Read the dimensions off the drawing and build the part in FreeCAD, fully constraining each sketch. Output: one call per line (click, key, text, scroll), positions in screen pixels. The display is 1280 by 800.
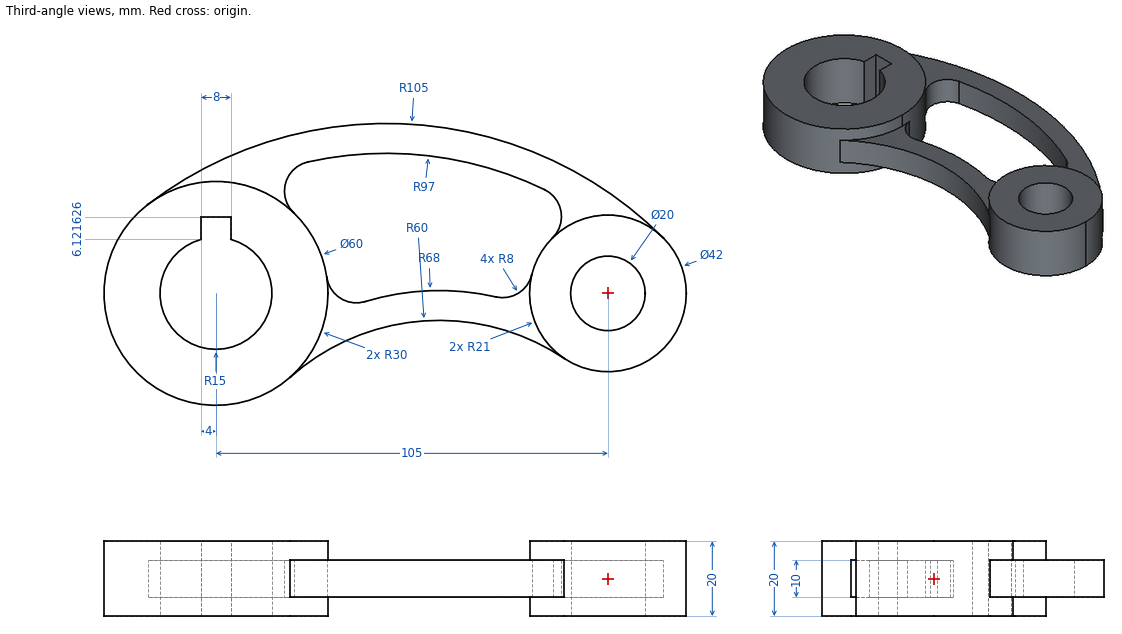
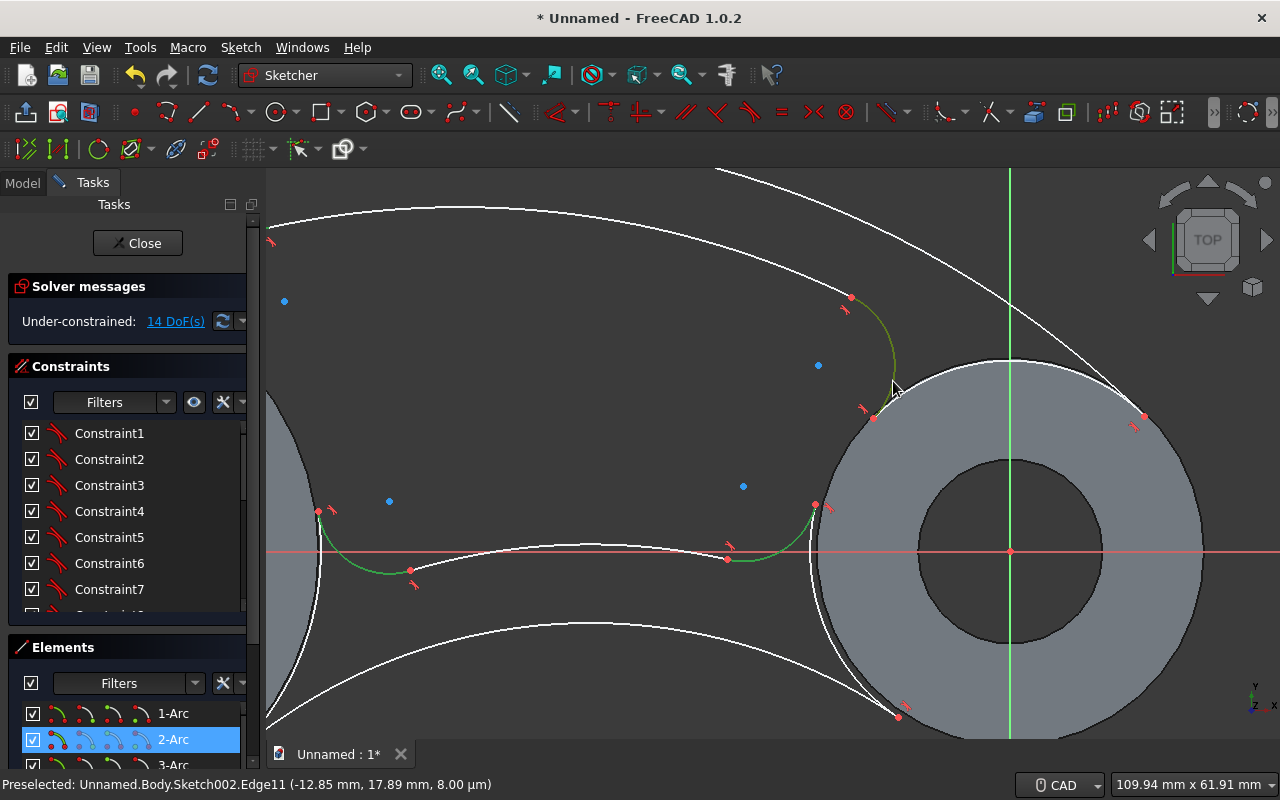
key(e)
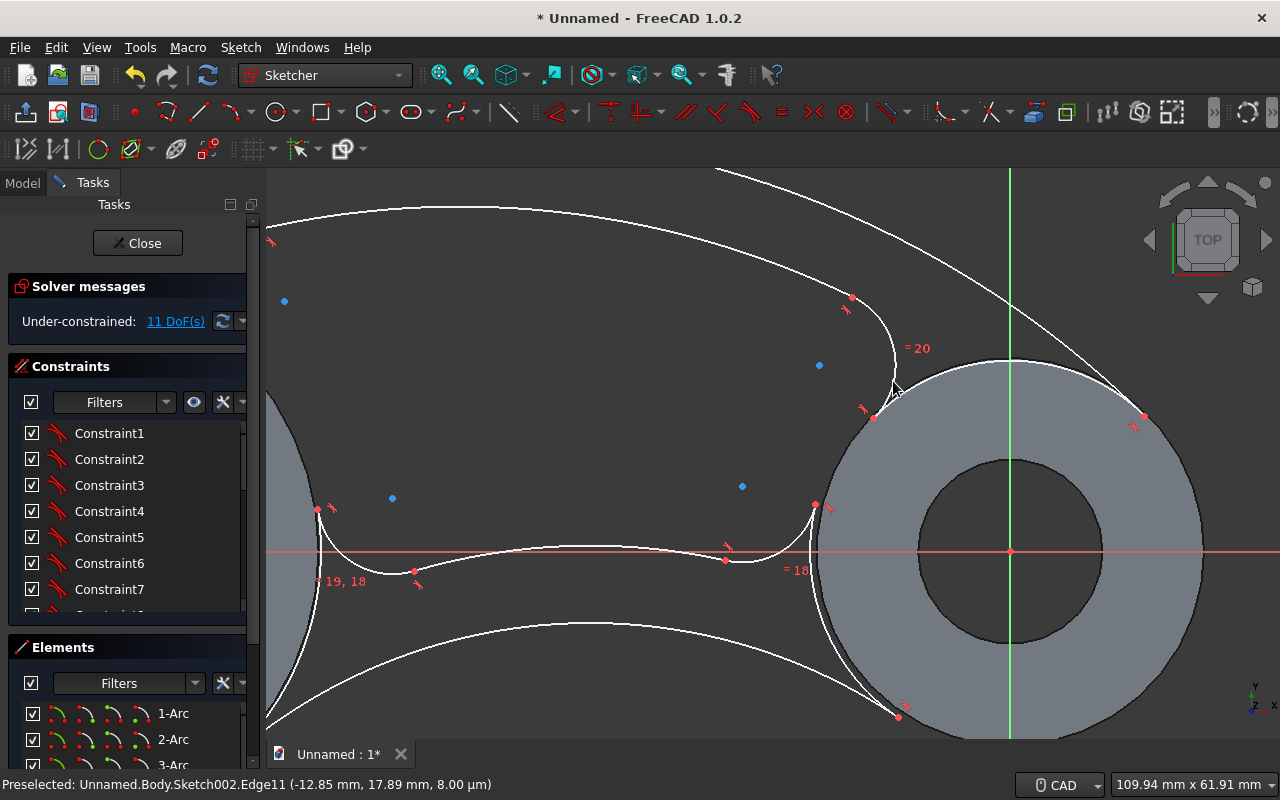
click(812, 577)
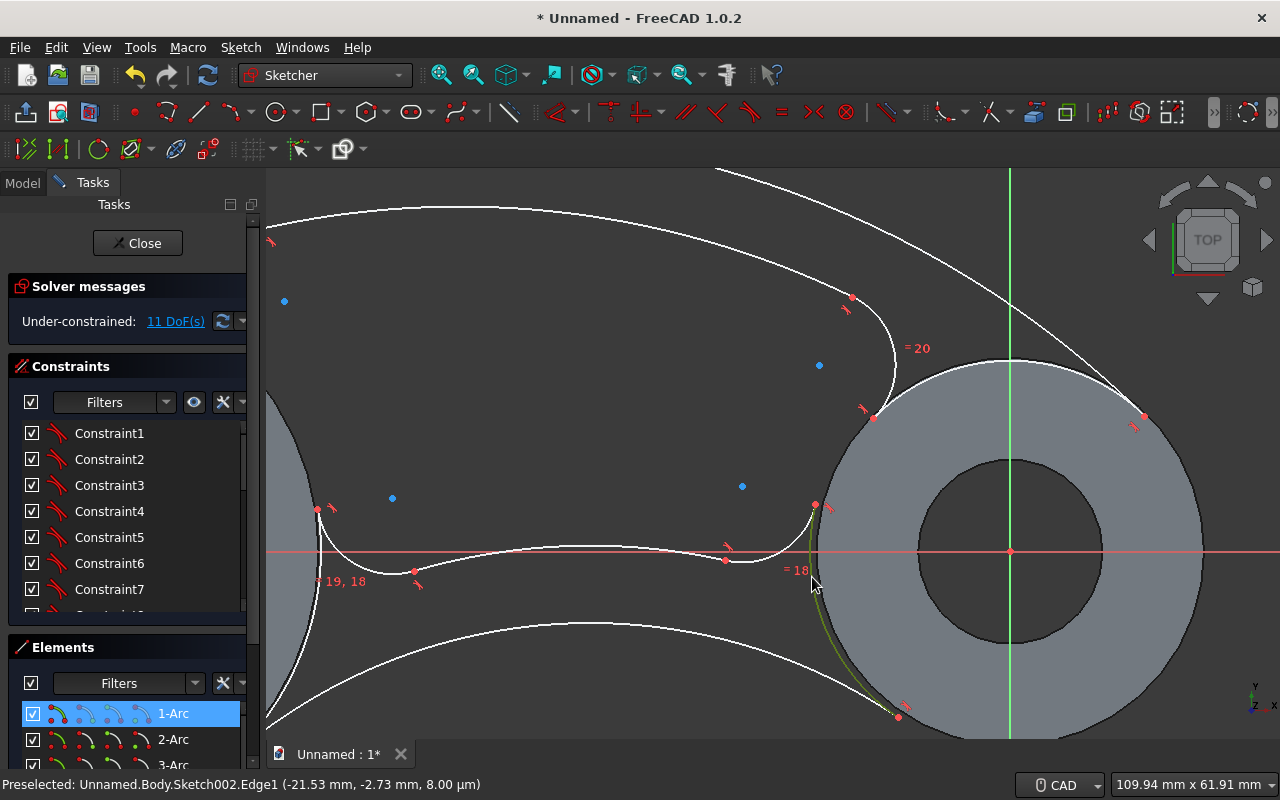
click(1068, 370)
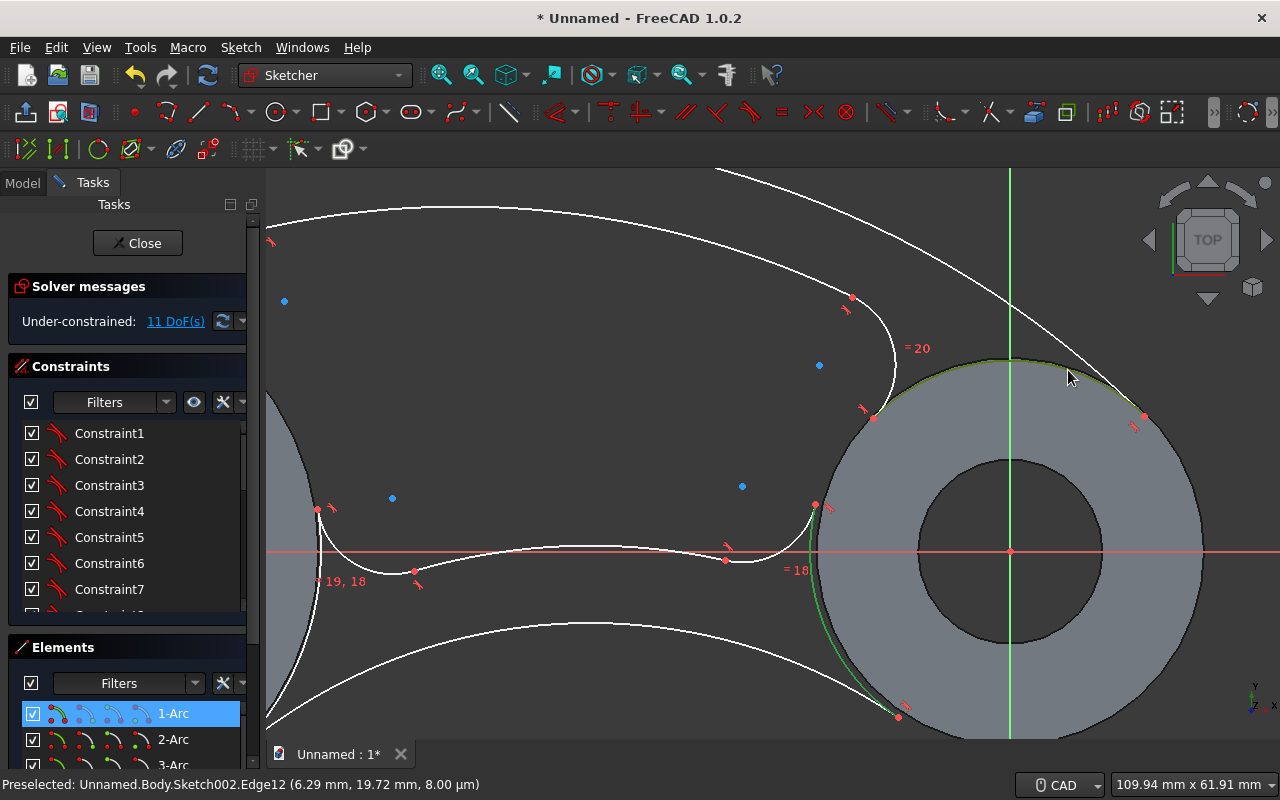
click(782, 112)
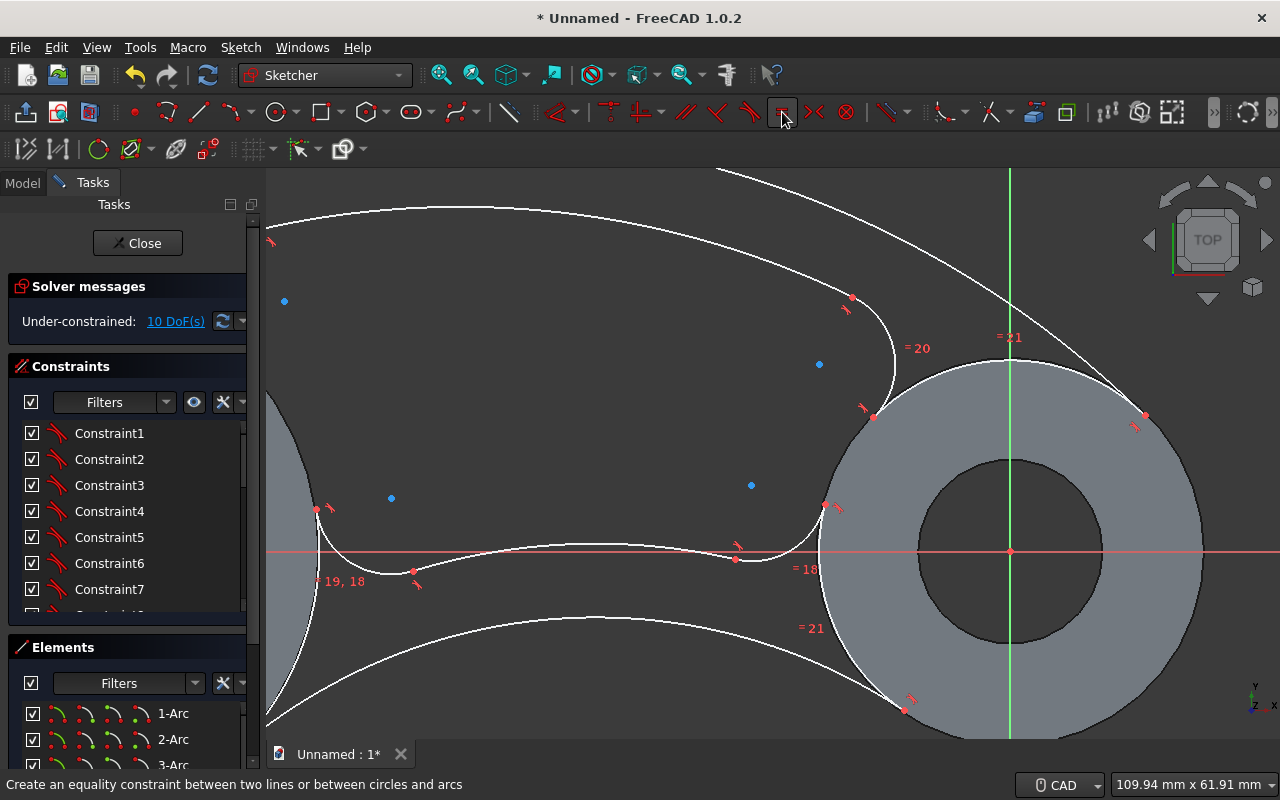
scroll(863, 460, down, 4)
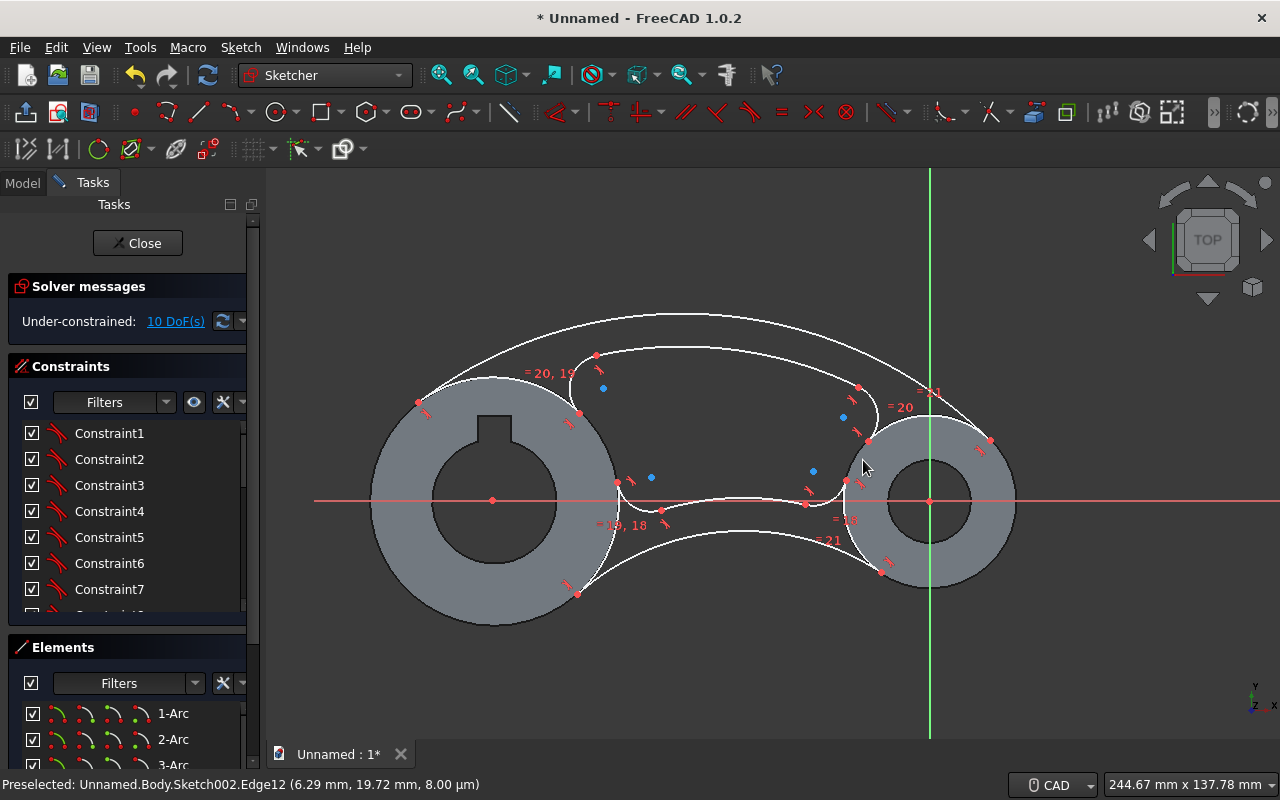
click(493, 501)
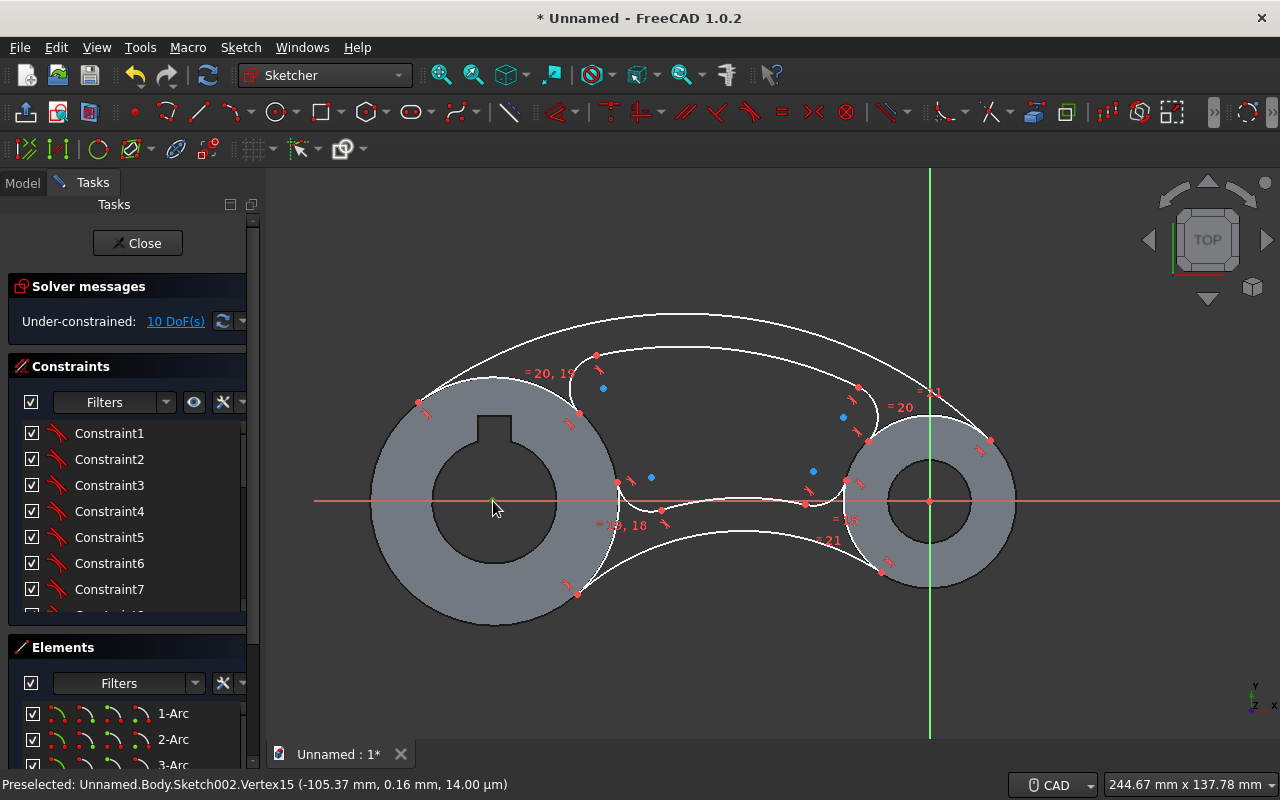
click(353, 501)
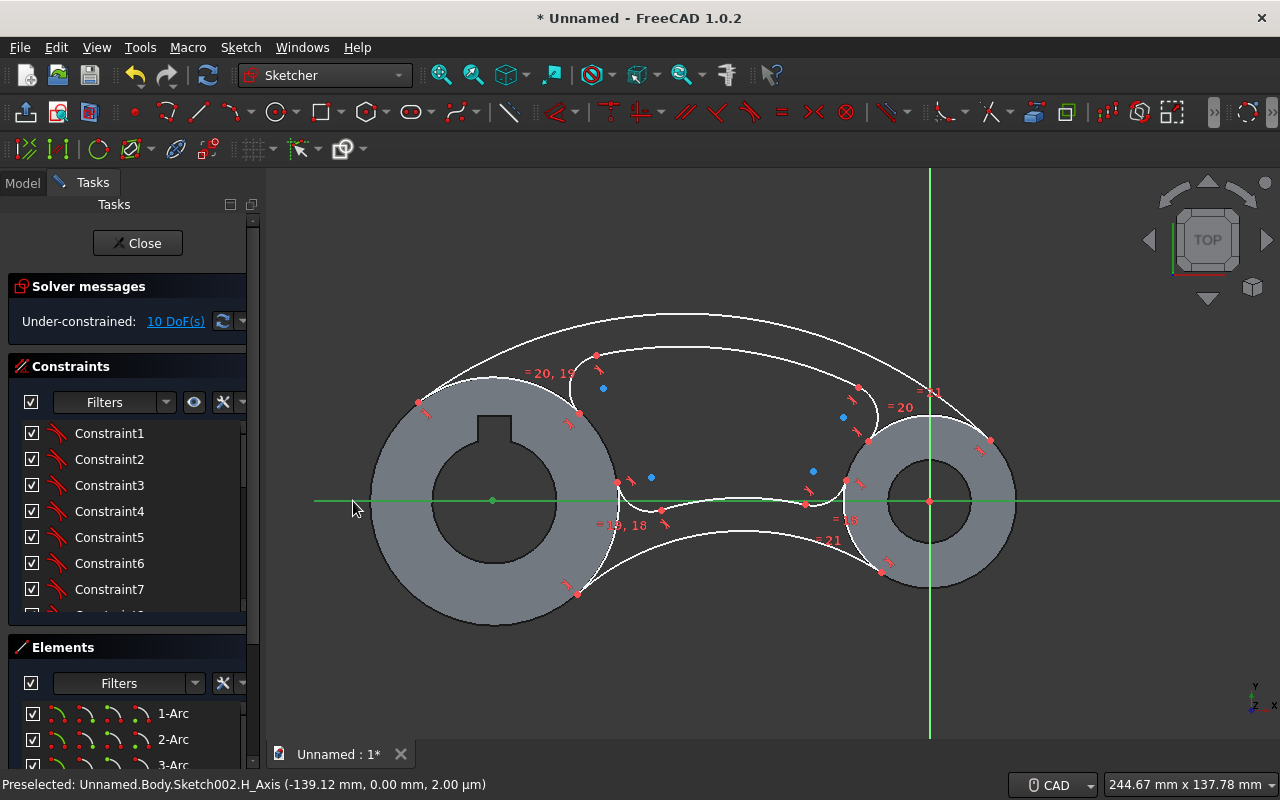
click(610, 112)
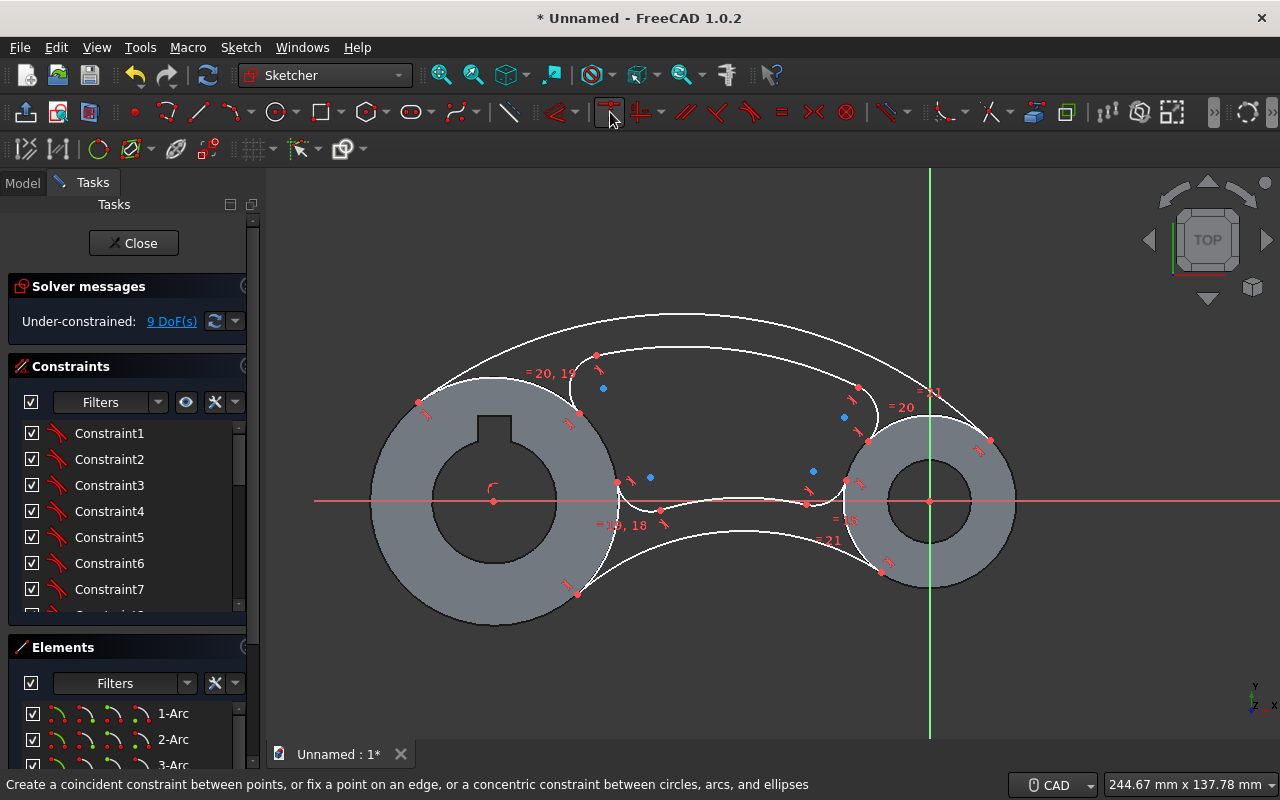
key(d)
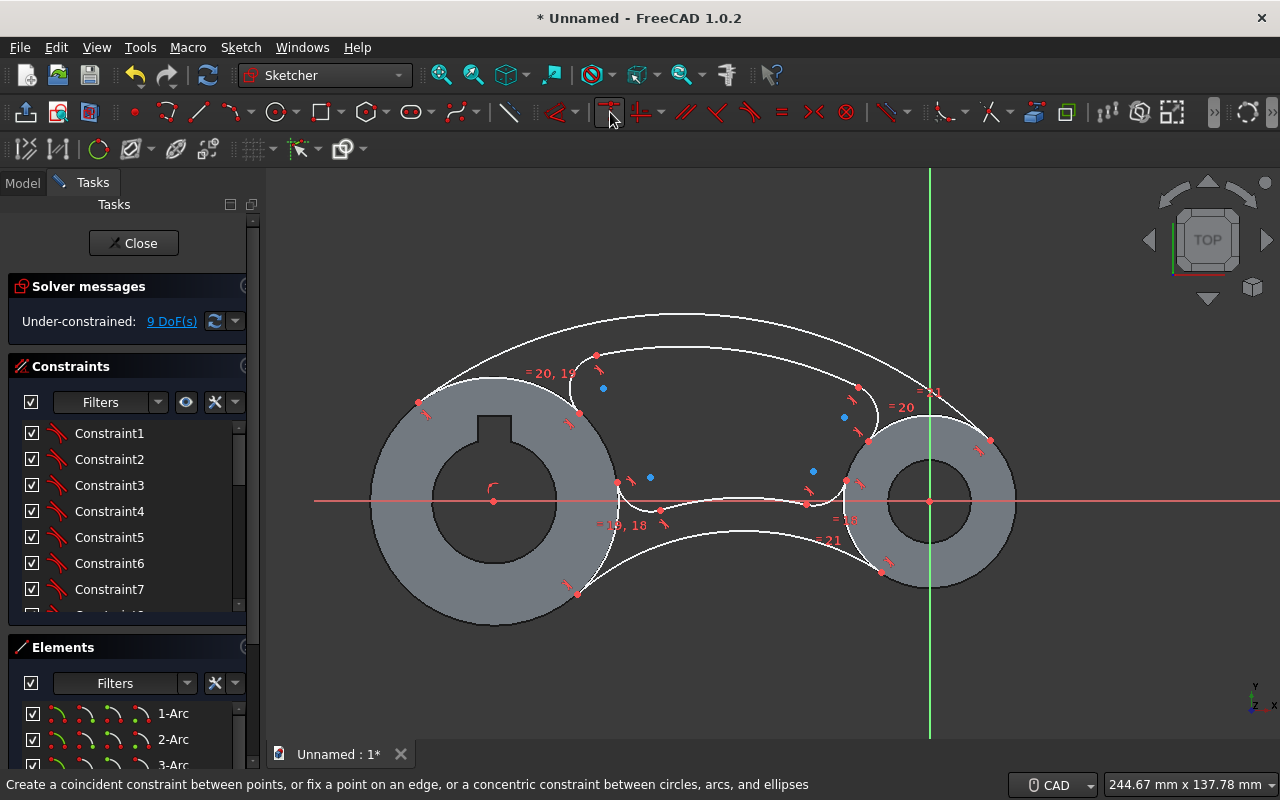
scroll(844, 512, up, 2)